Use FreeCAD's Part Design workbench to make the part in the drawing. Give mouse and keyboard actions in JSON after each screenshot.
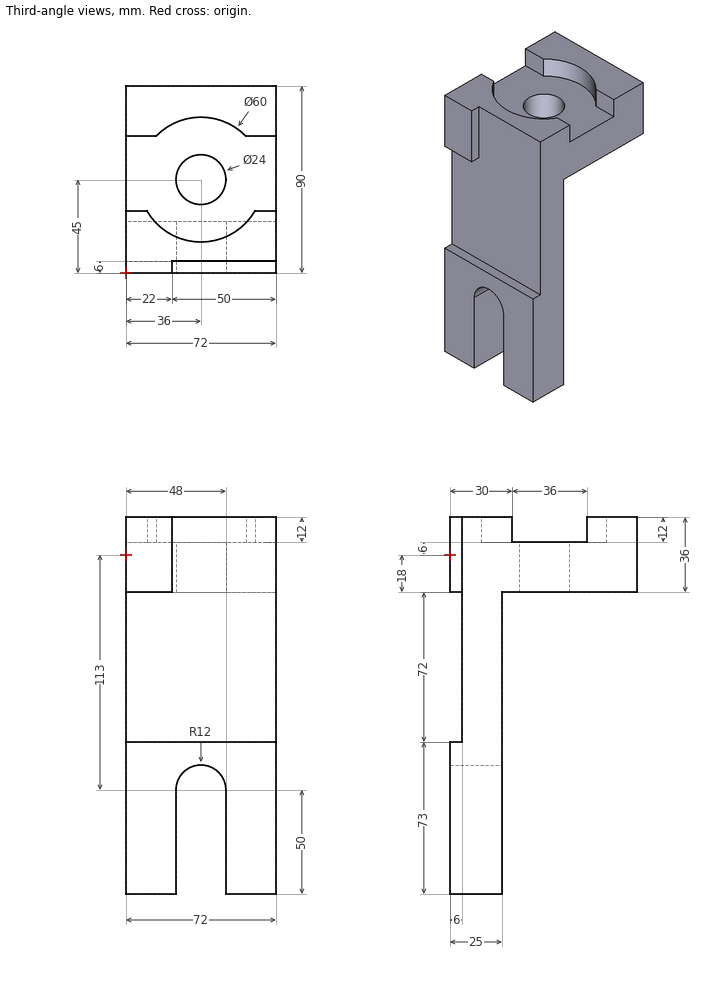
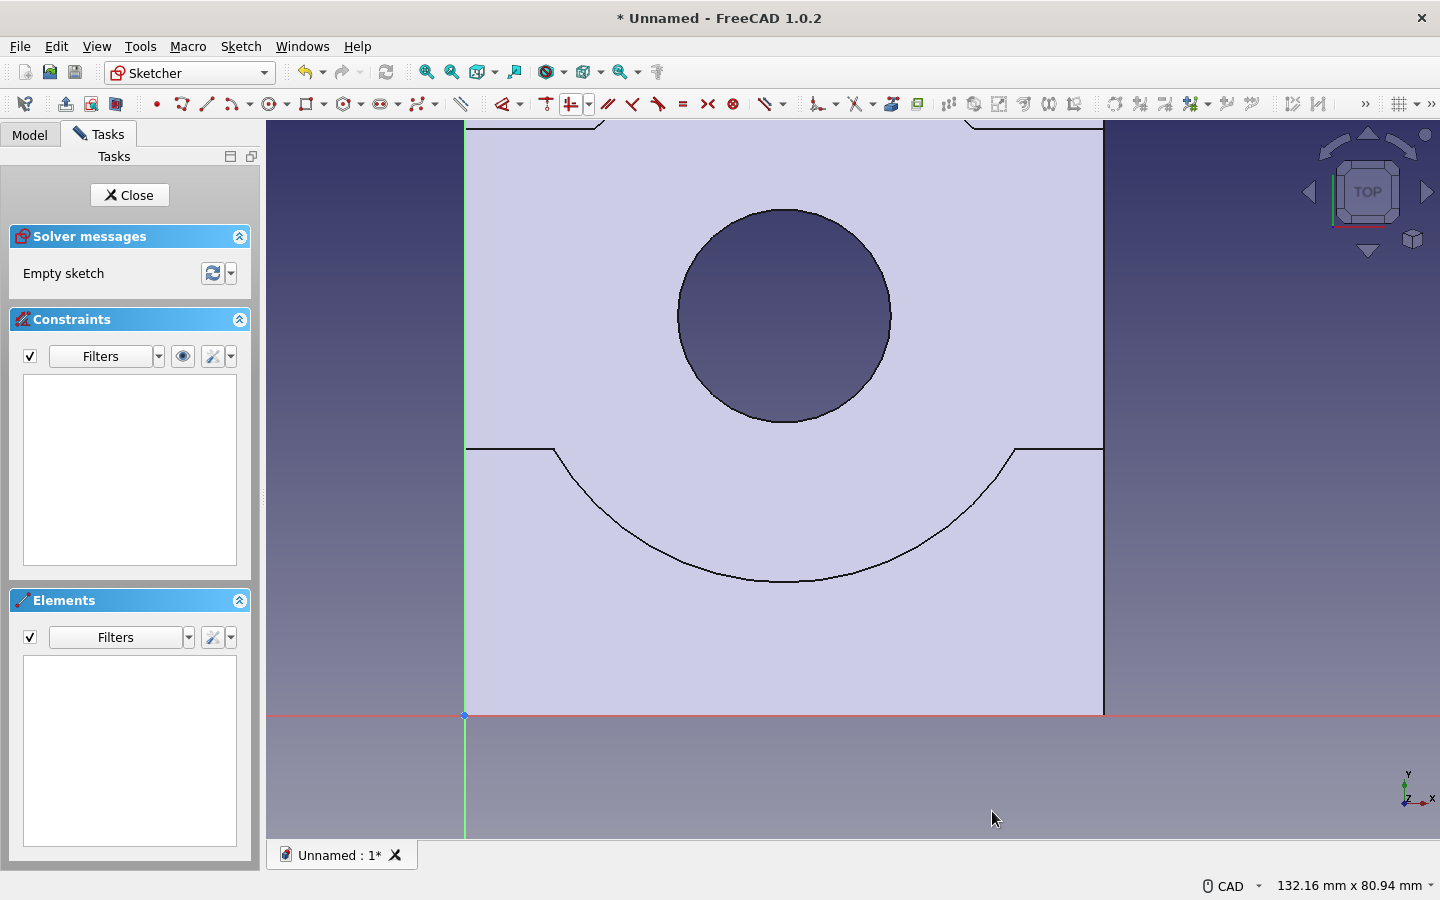
{"action": "key", "text": "g r"}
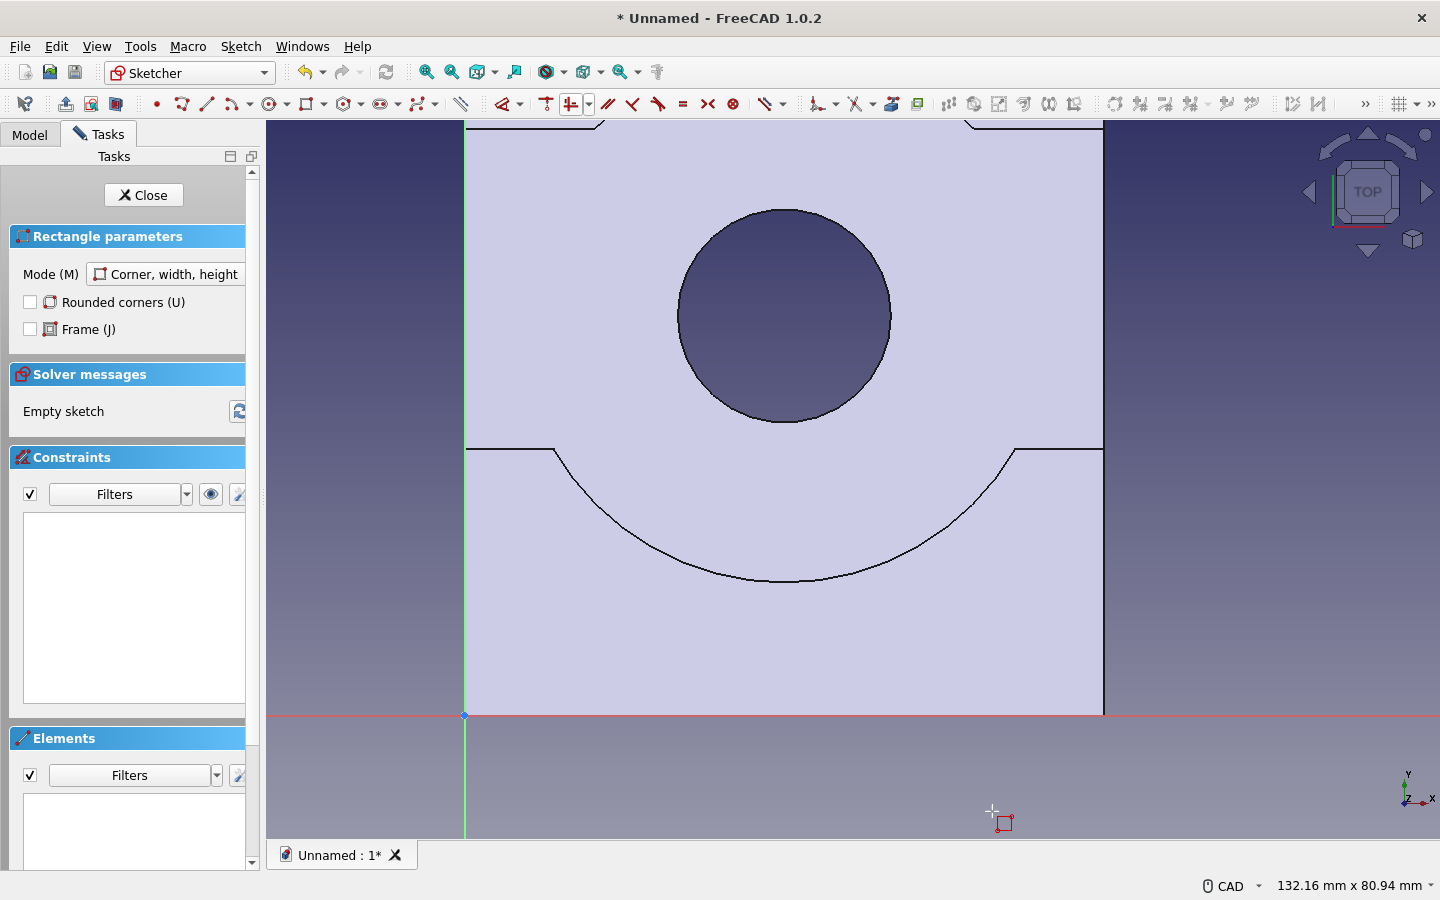
{"action": "left_click", "coordinate": [660, 662]}
{"action": "left_click", "coordinate": [1104, 716]}
{"action": "key", "text": "Escape"}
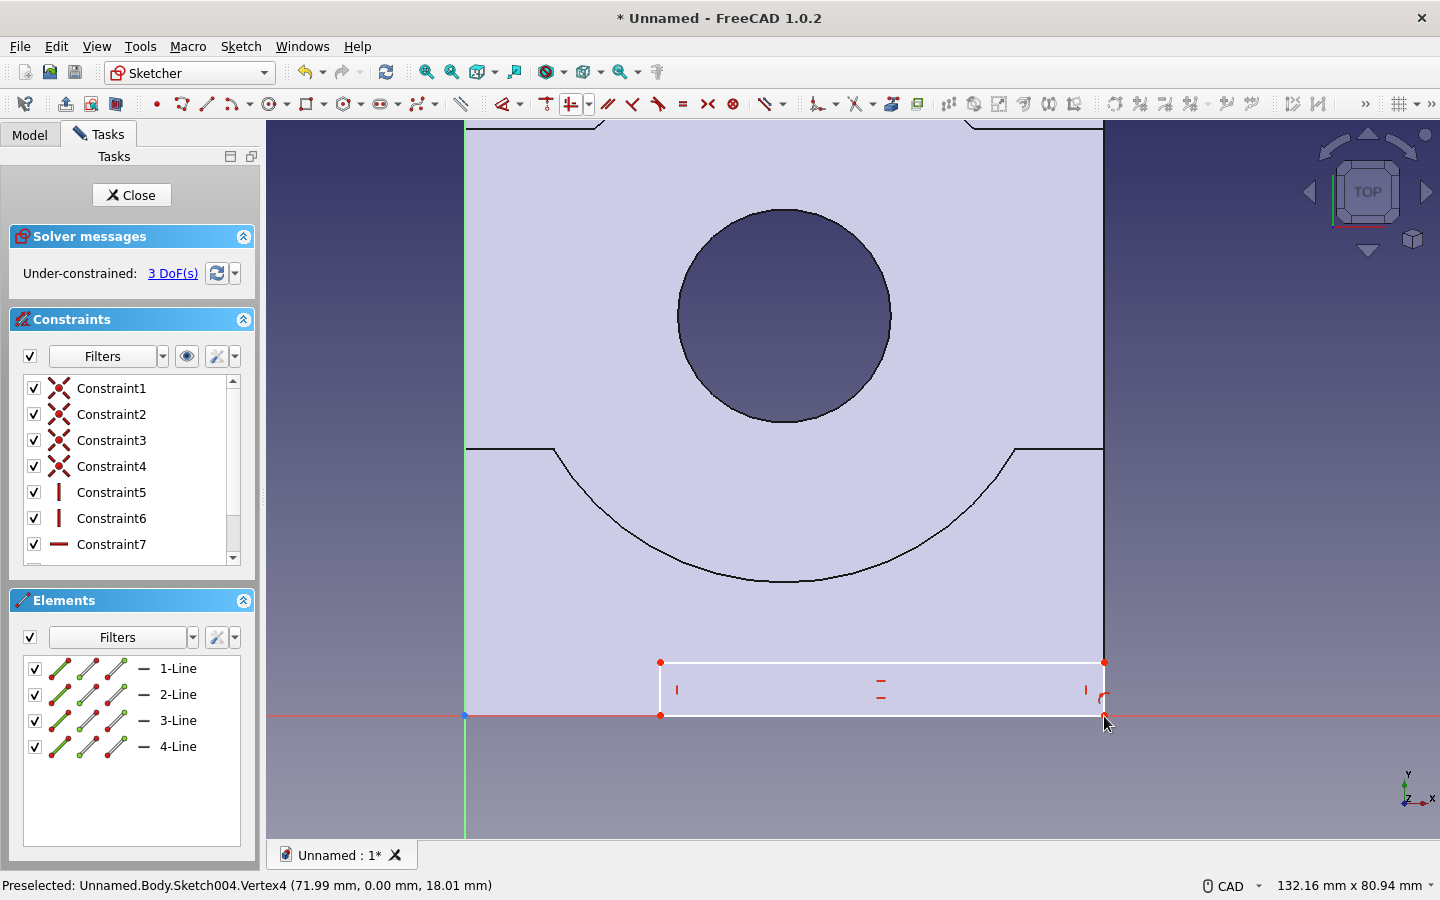
{"action": "left_click", "coordinate": [502, 104]}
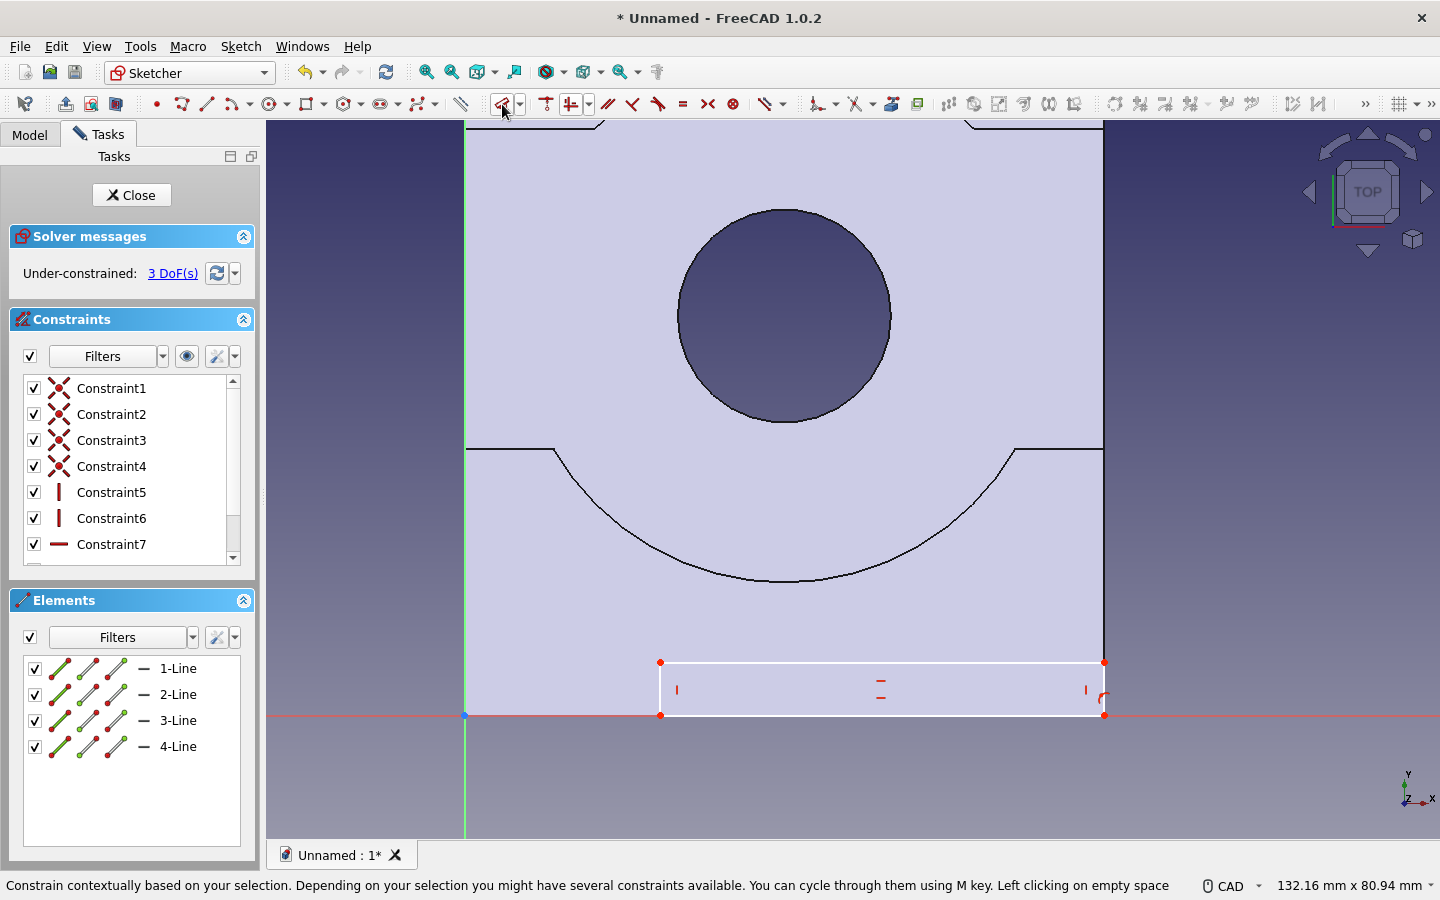
{"action": "left_click", "coordinate": [660, 679]}
{"action": "left_click", "coordinate": [626, 689]}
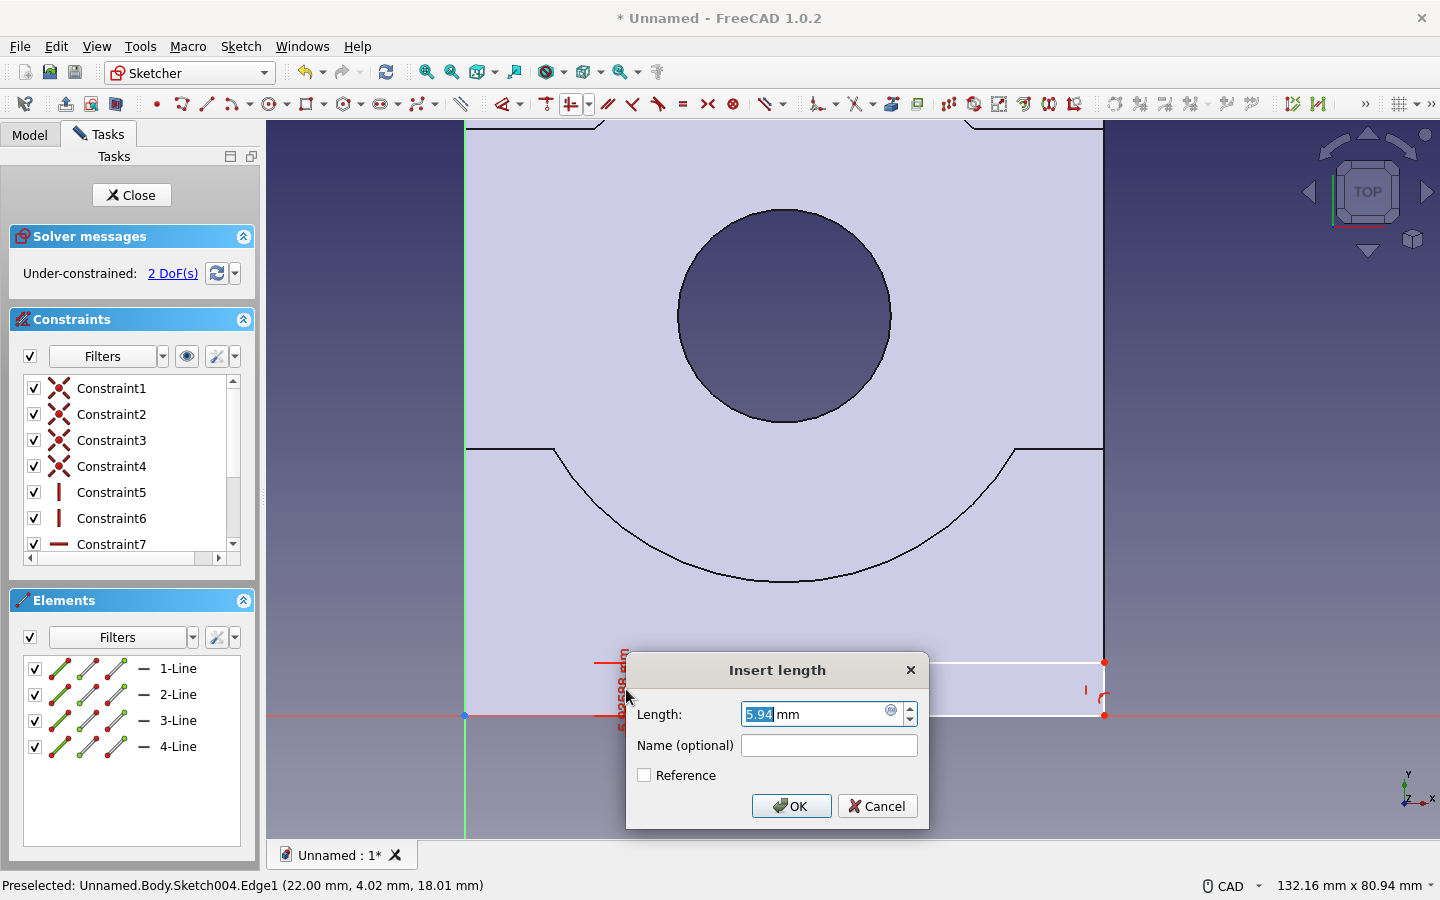
{"action": "type", "text": "6"}
{"action": "key", "text": "Return"}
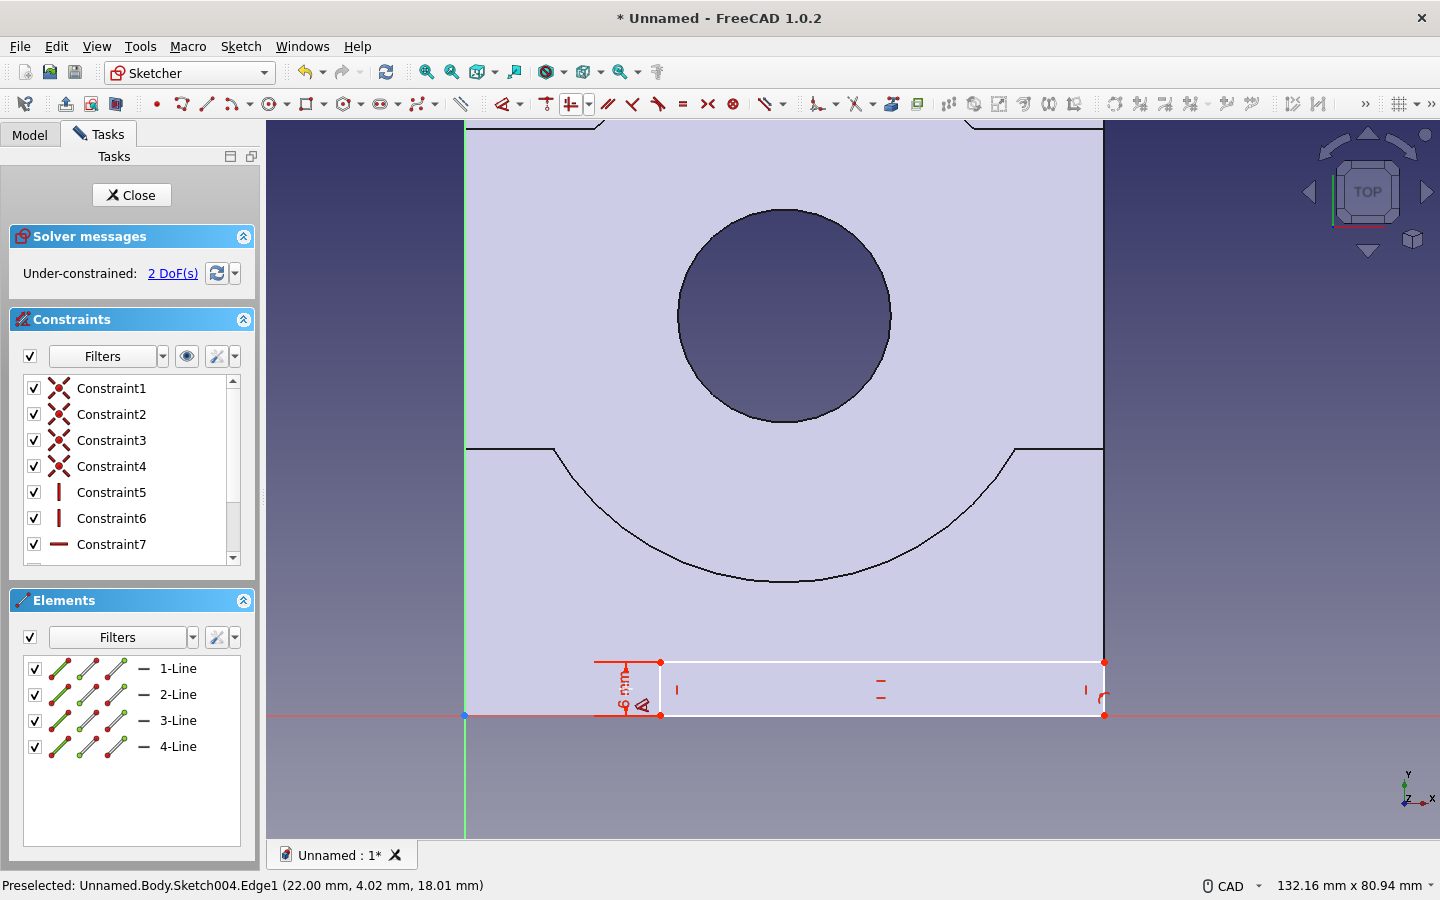
{"action": "left_click", "coordinate": [793, 716]}
{"action": "left_click", "coordinate": [882, 750]}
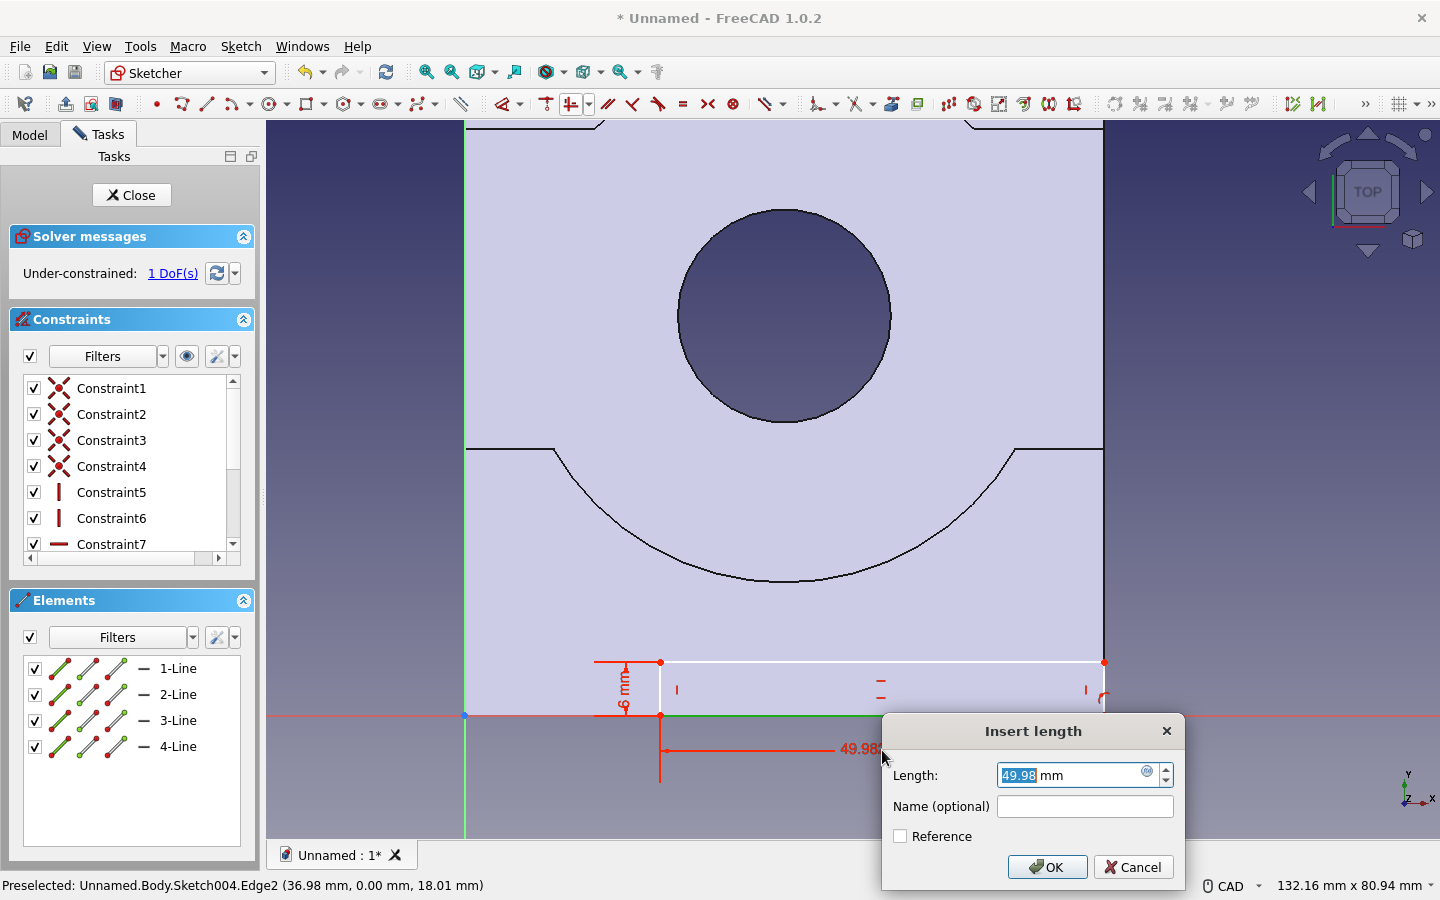
{"action": "type", "text": "50"}
{"action": "key", "text": "Return"}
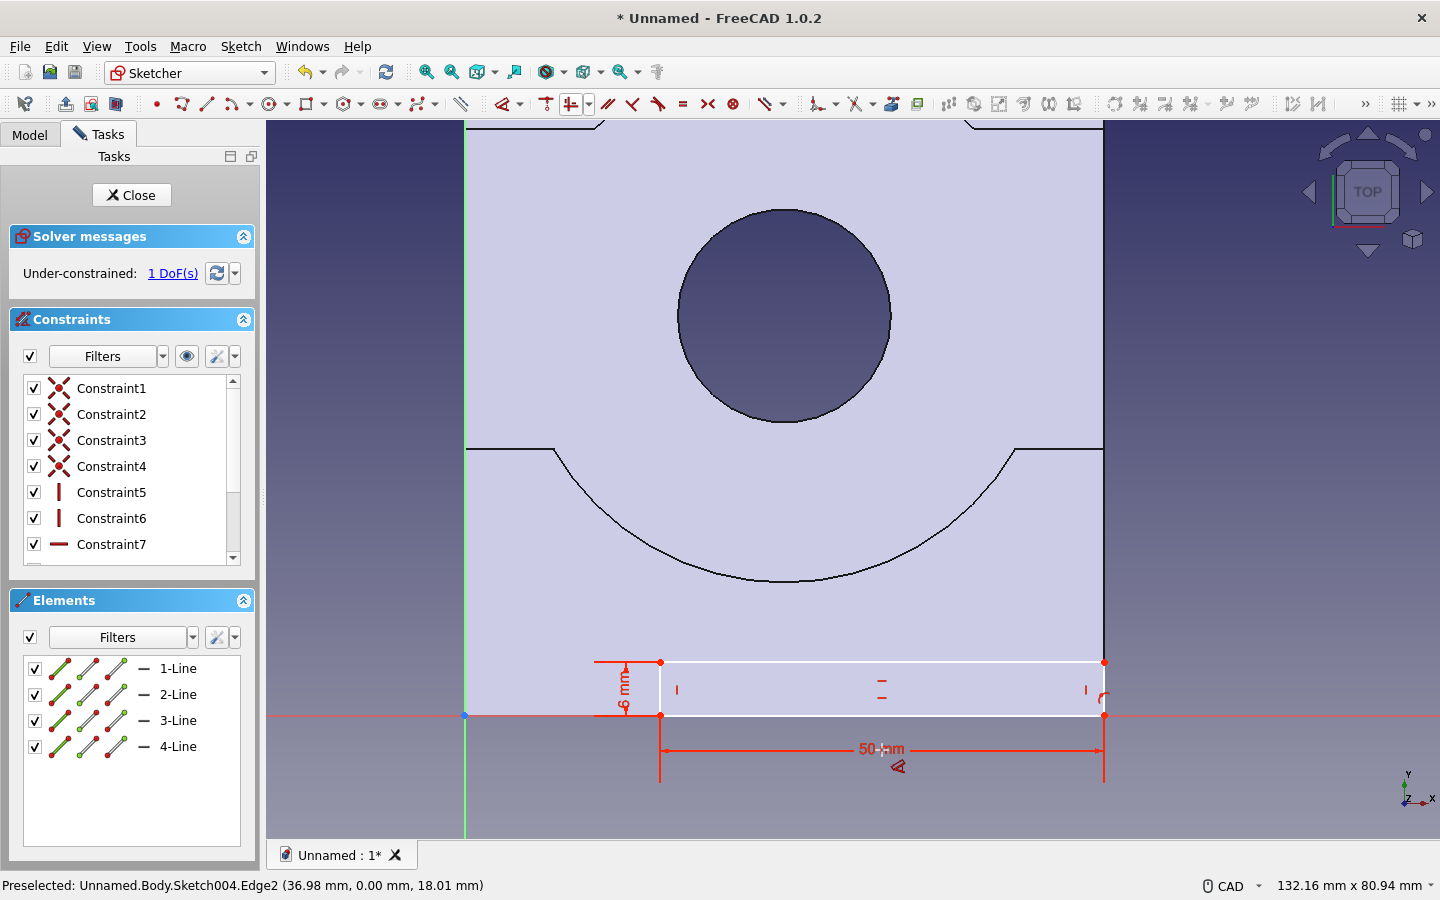
{"action": "left_click", "coordinate": [660, 662]}
{"action": "left_click", "coordinate": [562, 750]}